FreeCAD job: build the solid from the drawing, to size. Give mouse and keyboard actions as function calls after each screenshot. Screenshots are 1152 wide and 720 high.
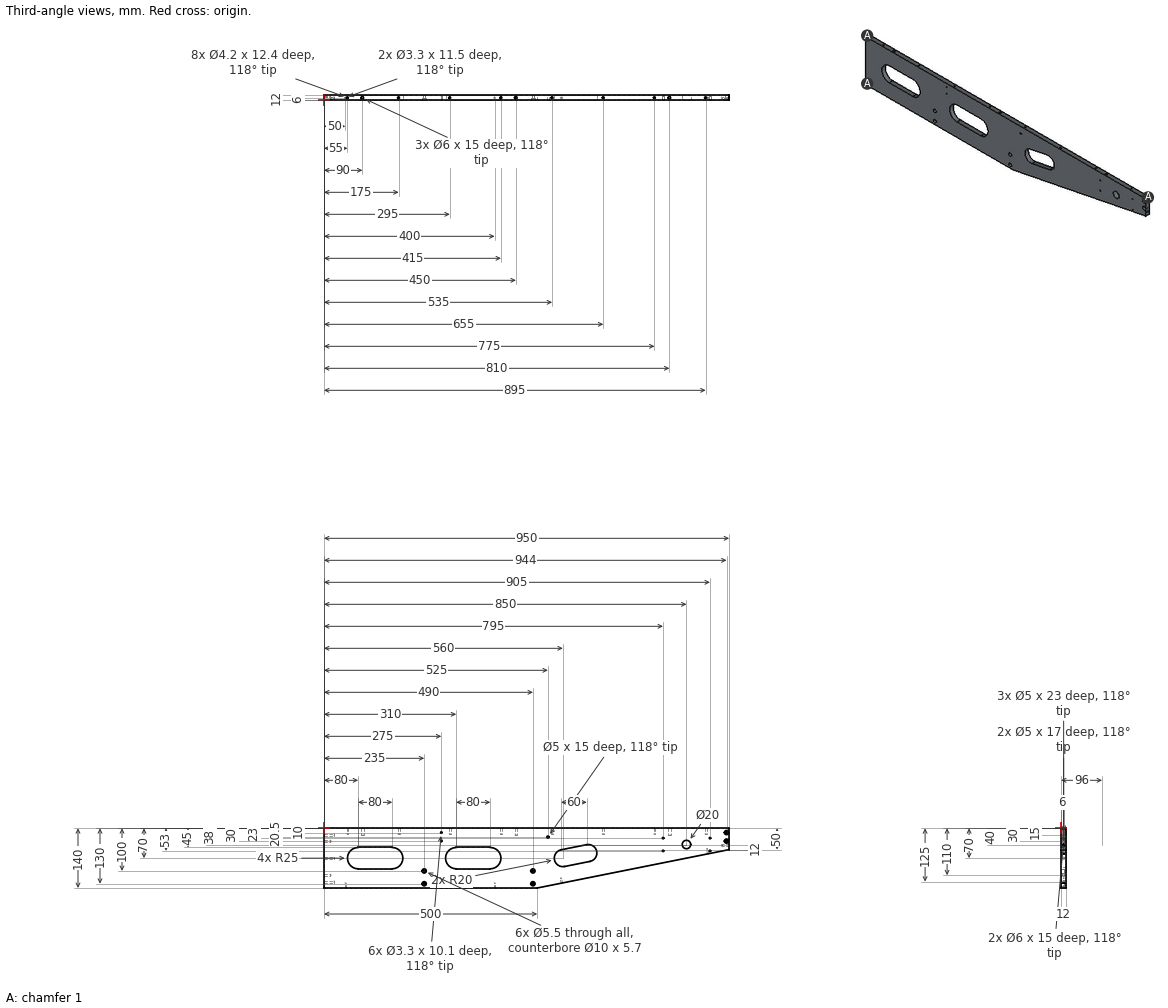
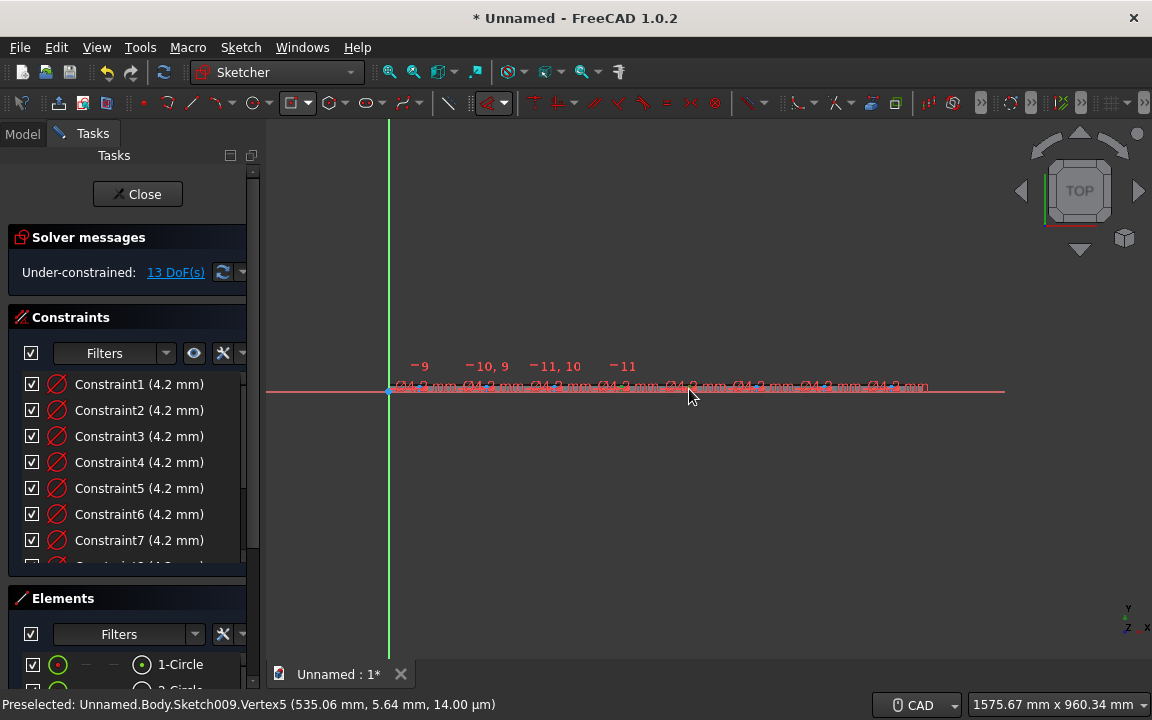
key(h)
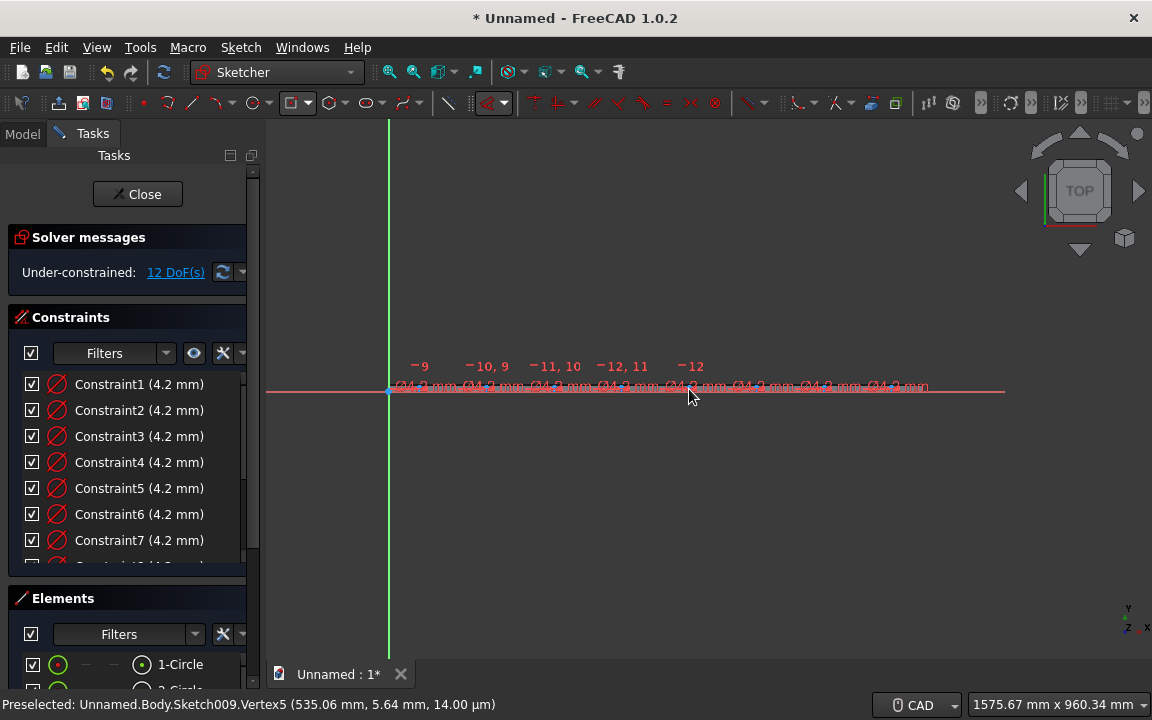
click(689, 389)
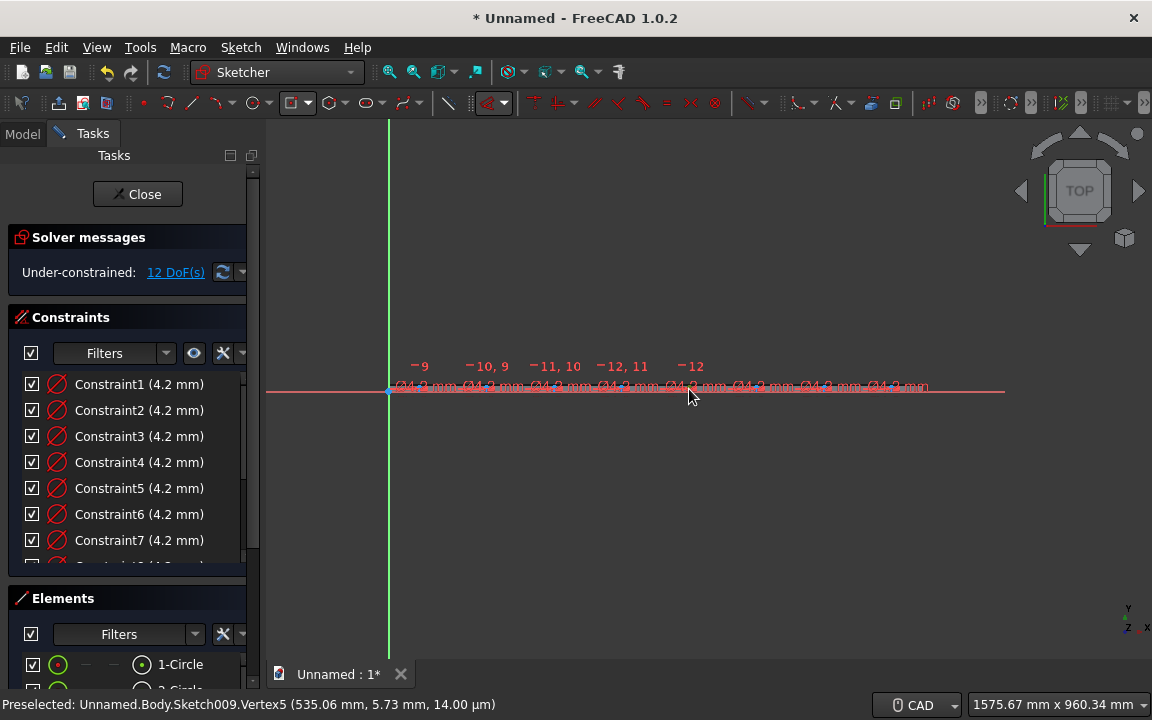
click(757, 389)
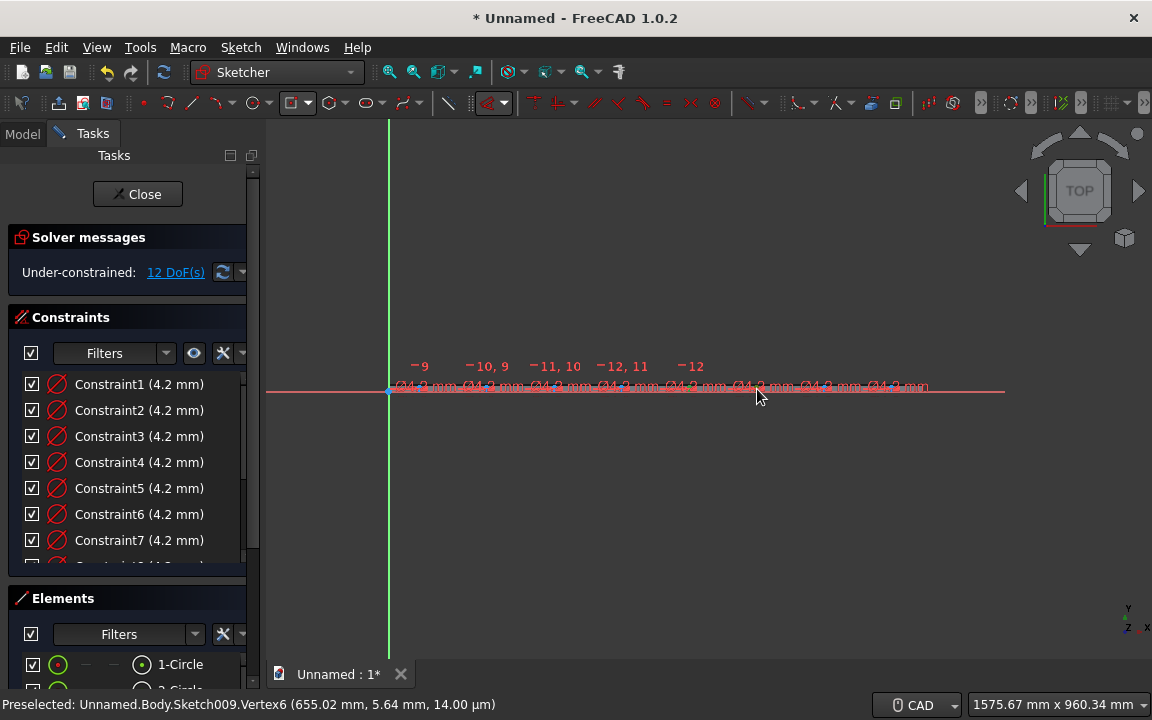
key(h)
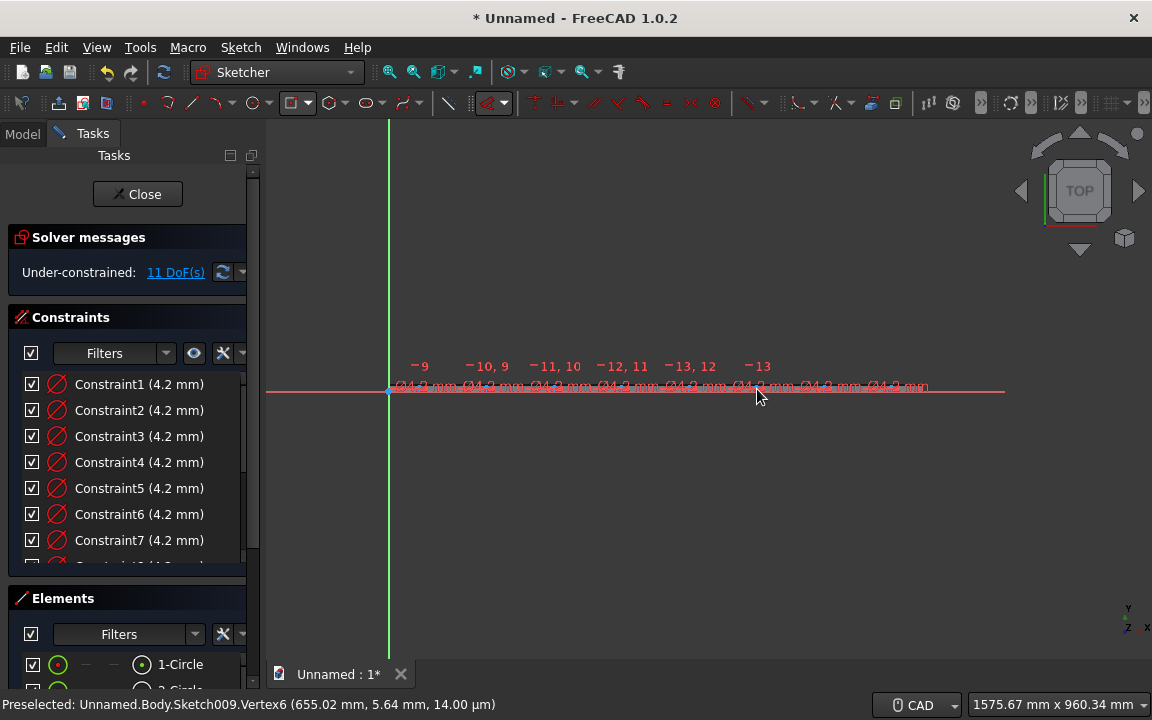
click(757, 389)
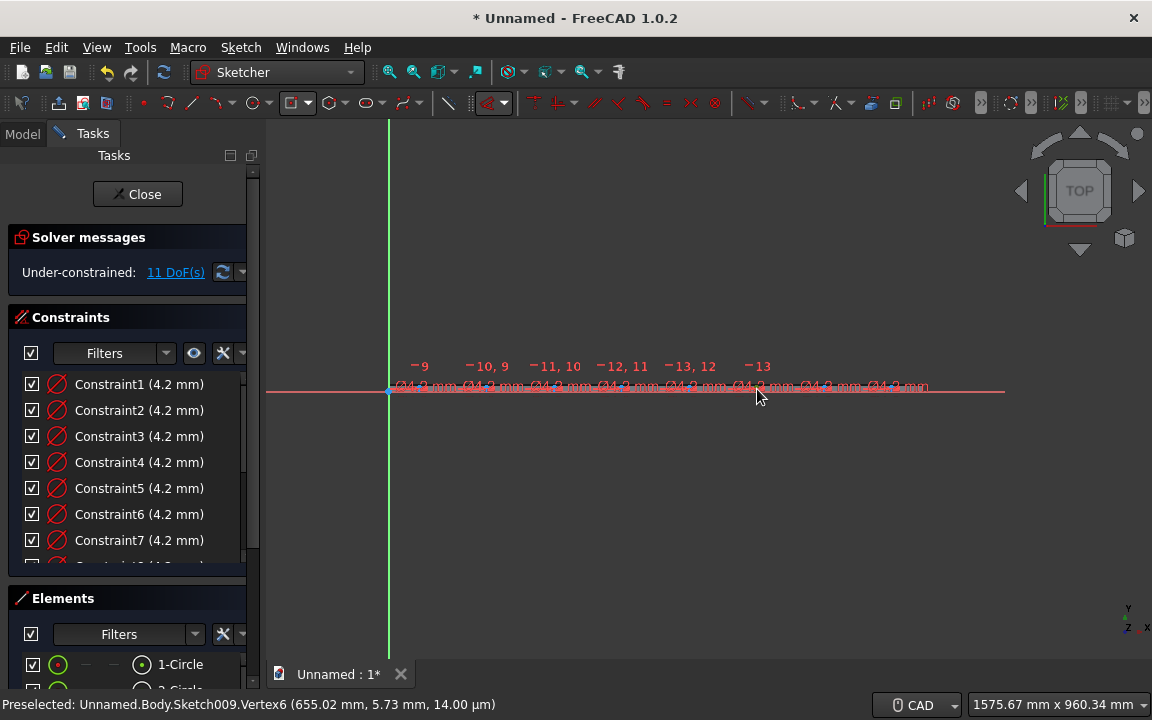
click(824, 389)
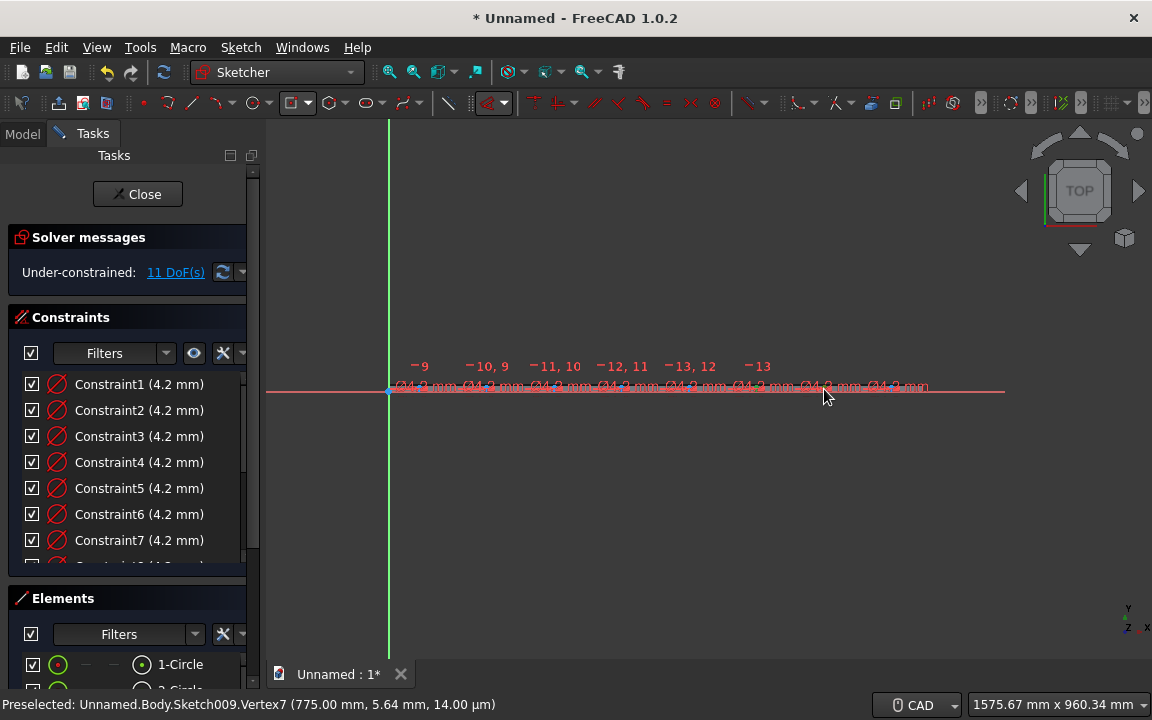
key(h)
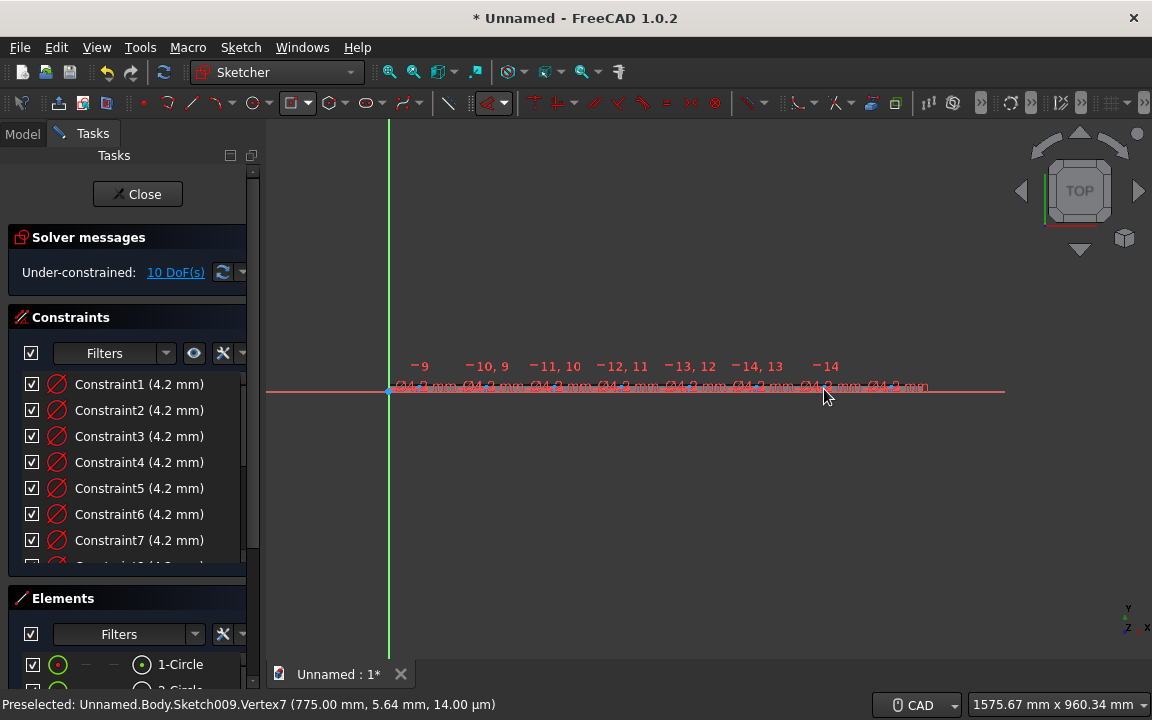
click(824, 389)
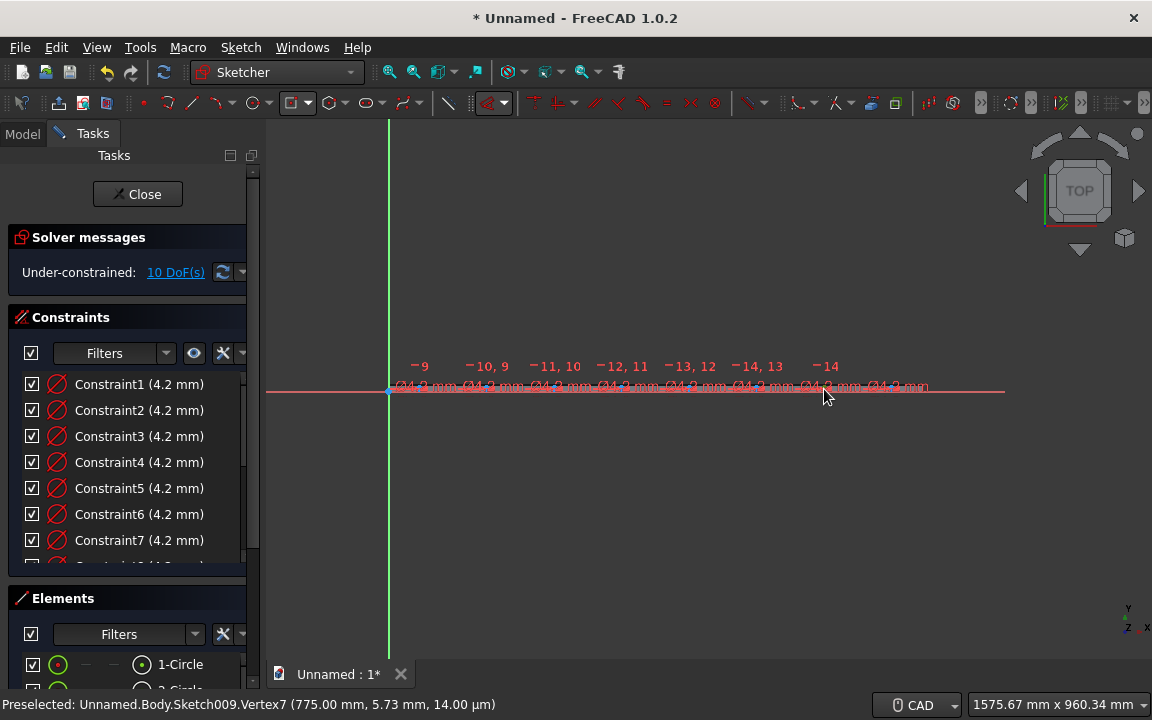
click(892, 389)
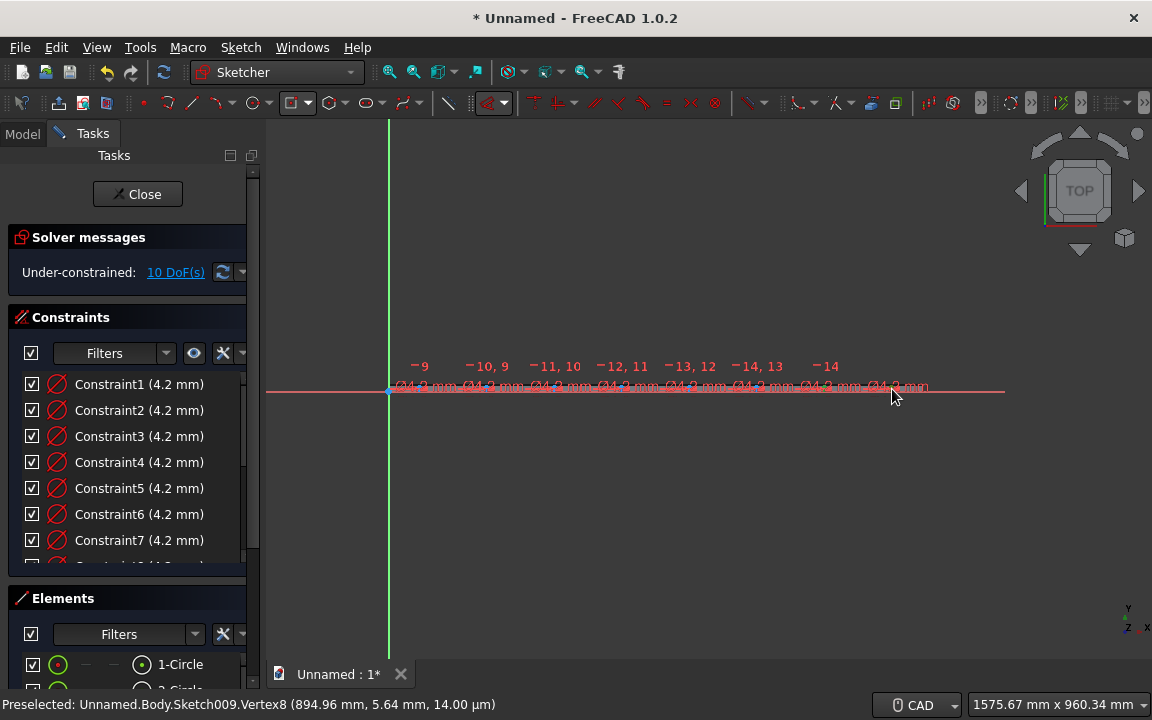
click(576, 104)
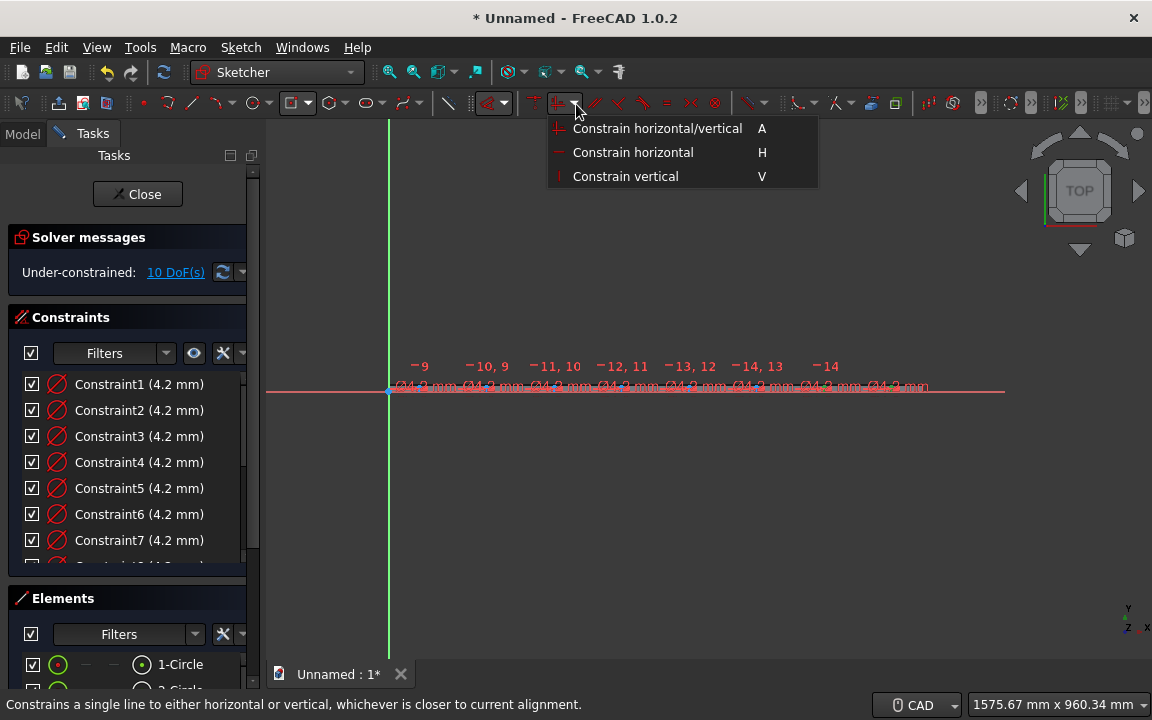
click(683, 152)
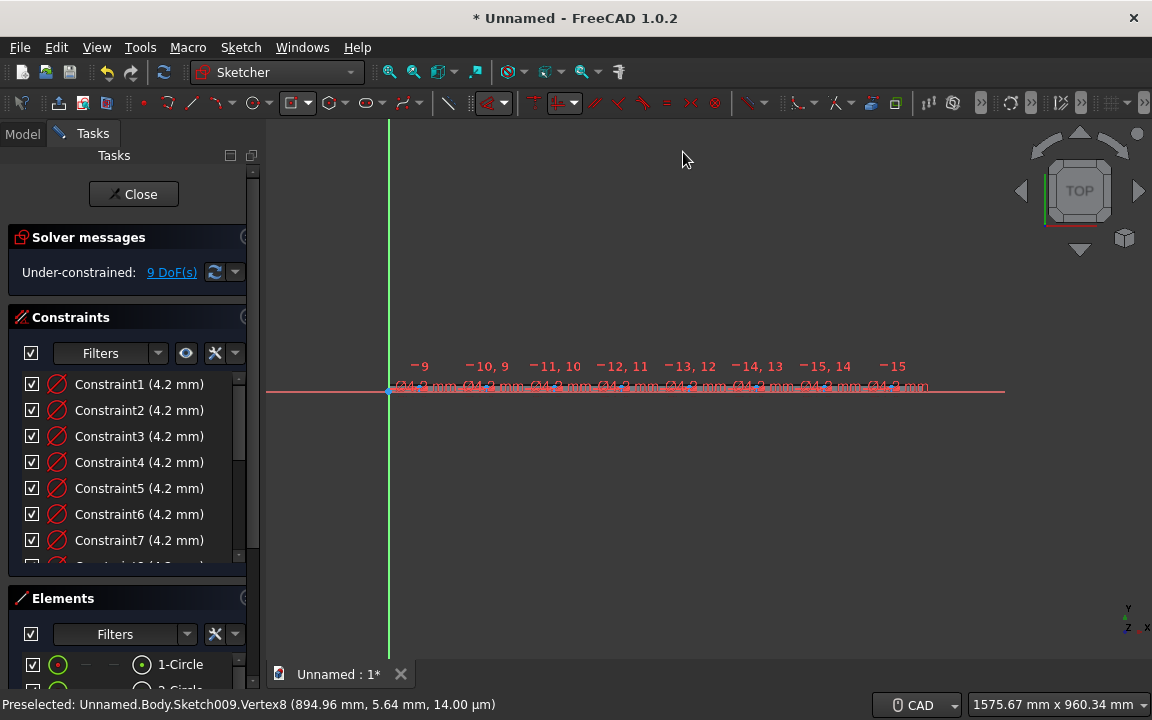
scroll(420, 389, up, 13)